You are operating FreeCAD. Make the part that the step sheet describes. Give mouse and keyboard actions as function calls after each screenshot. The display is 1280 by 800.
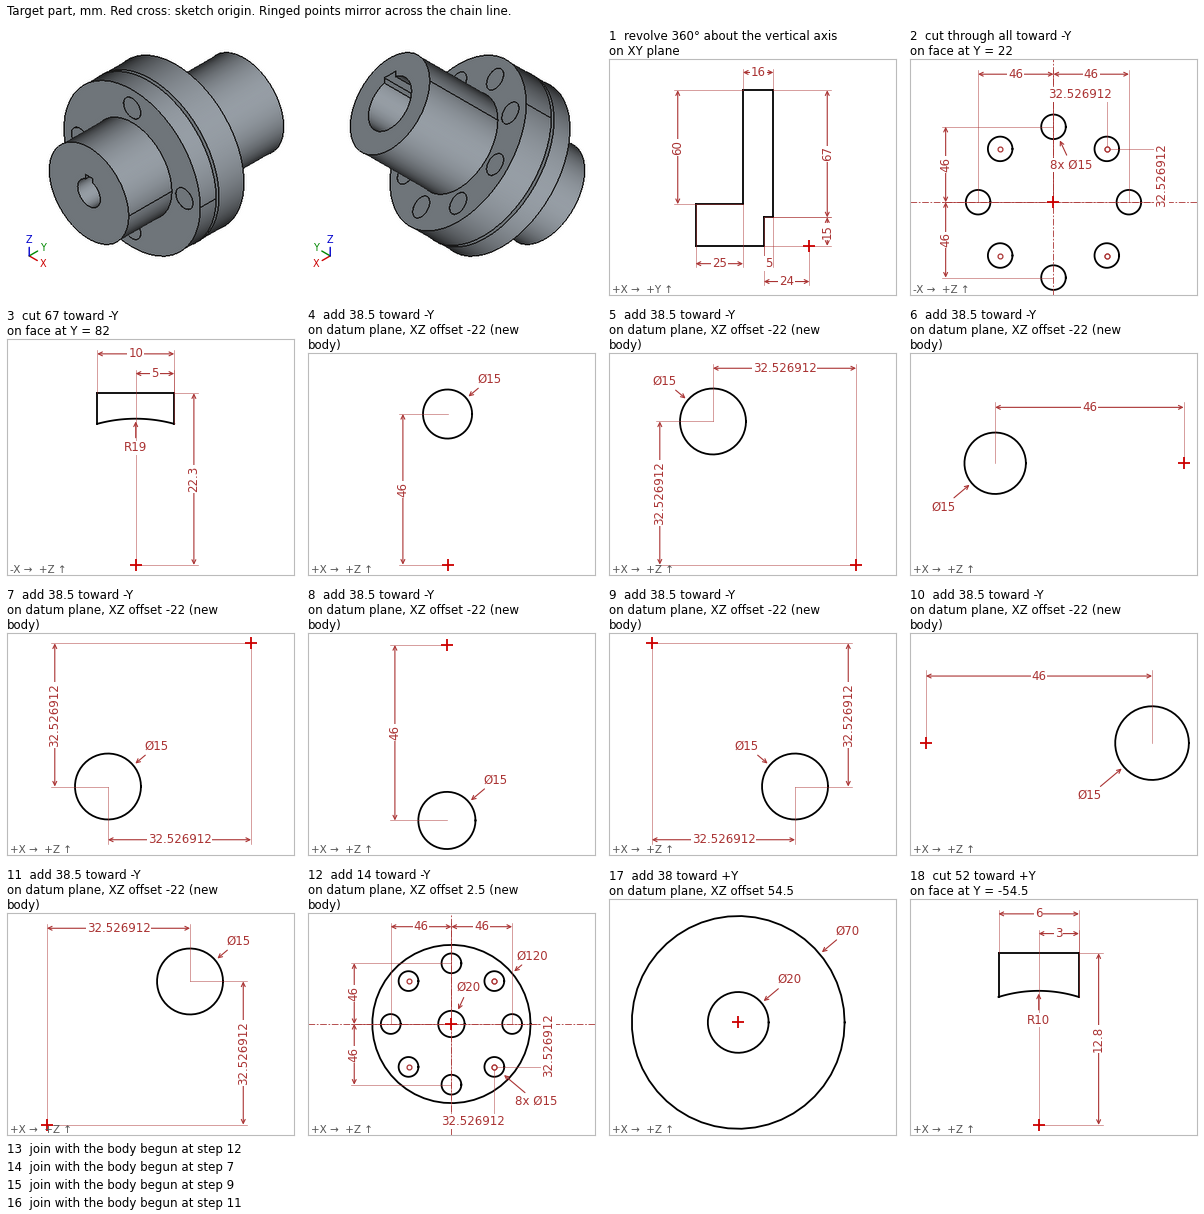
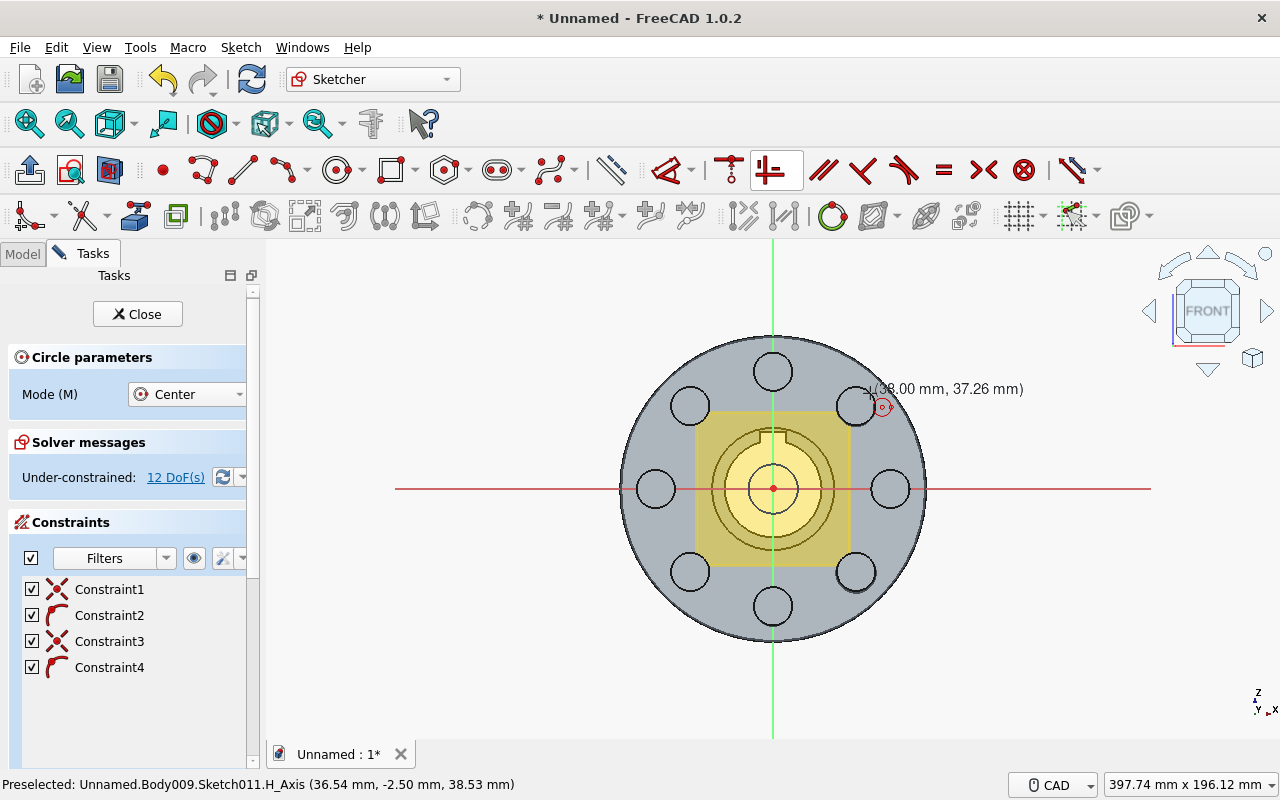
click(690, 572)
click(704, 558)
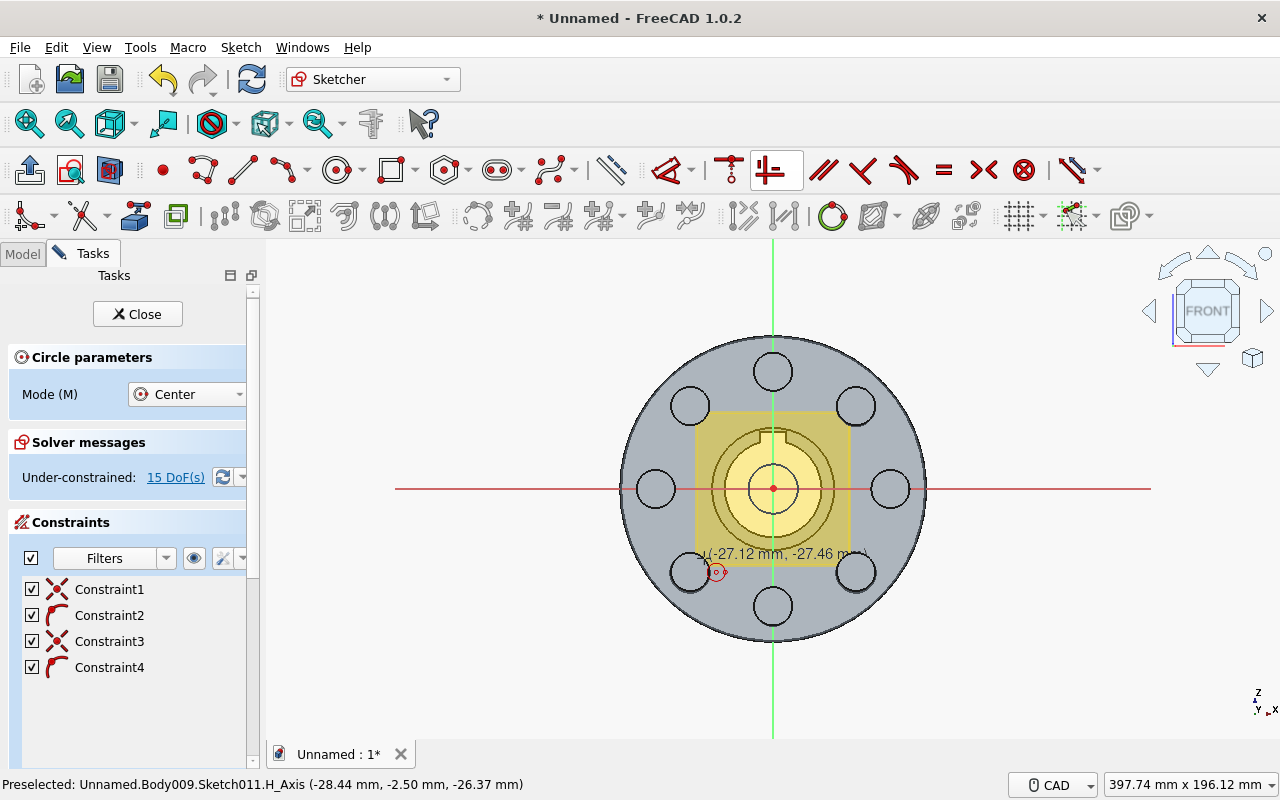
click(656, 489)
click(662, 471)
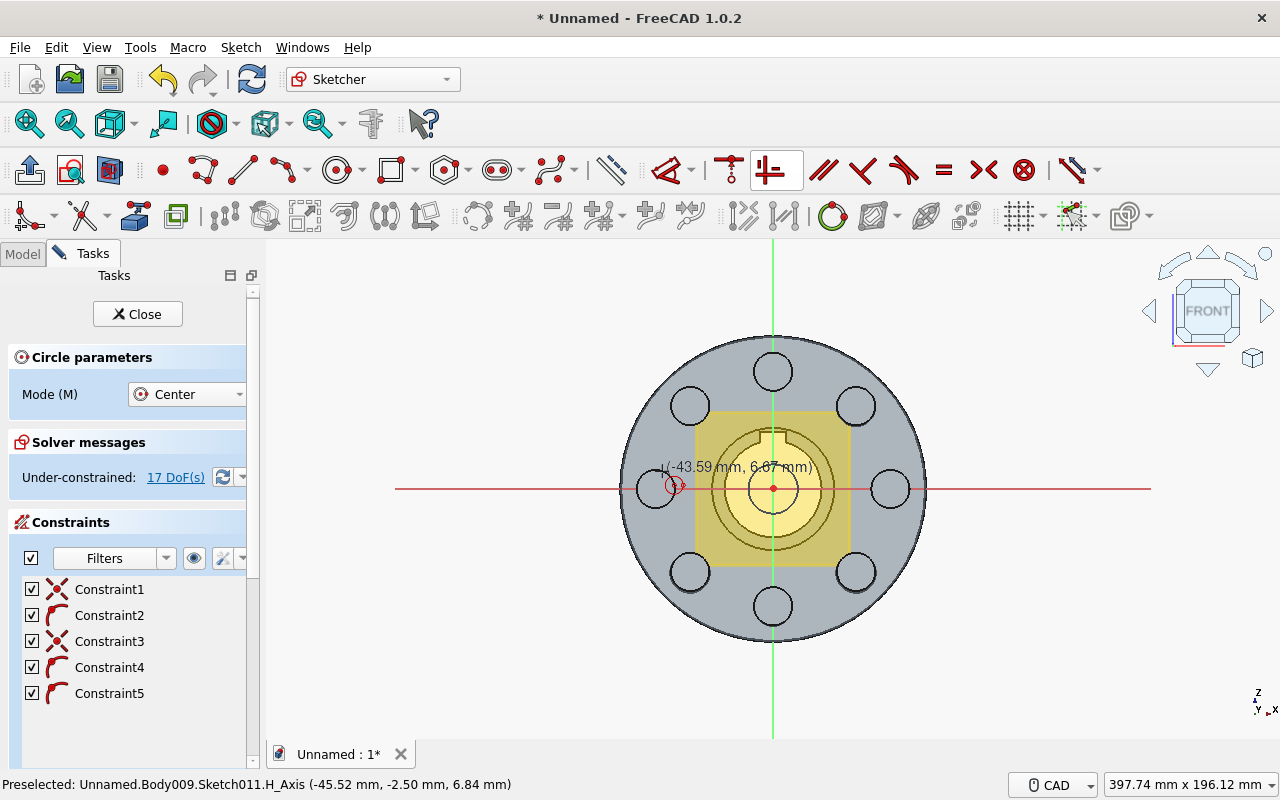
click(773, 372)
click(791, 365)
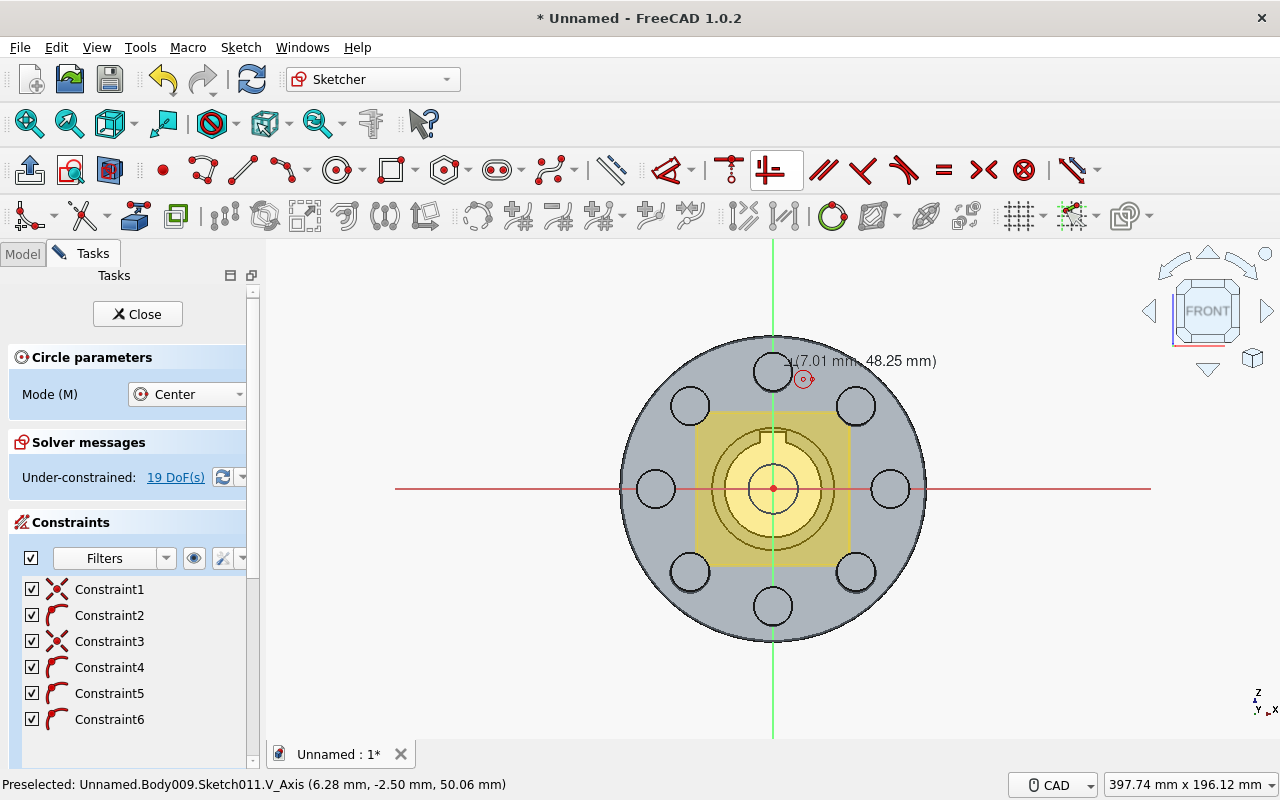
click(690, 406)
click(704, 393)
key(Escape)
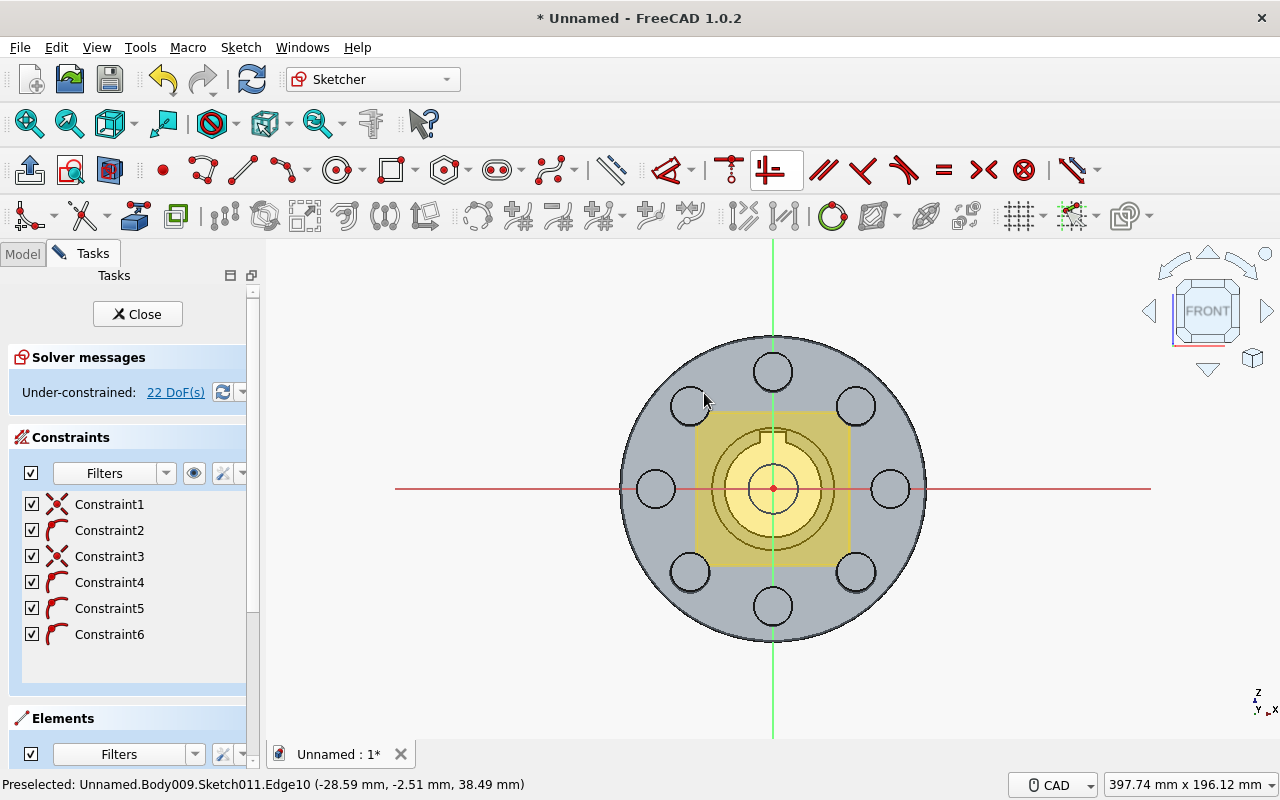
click(870, 559)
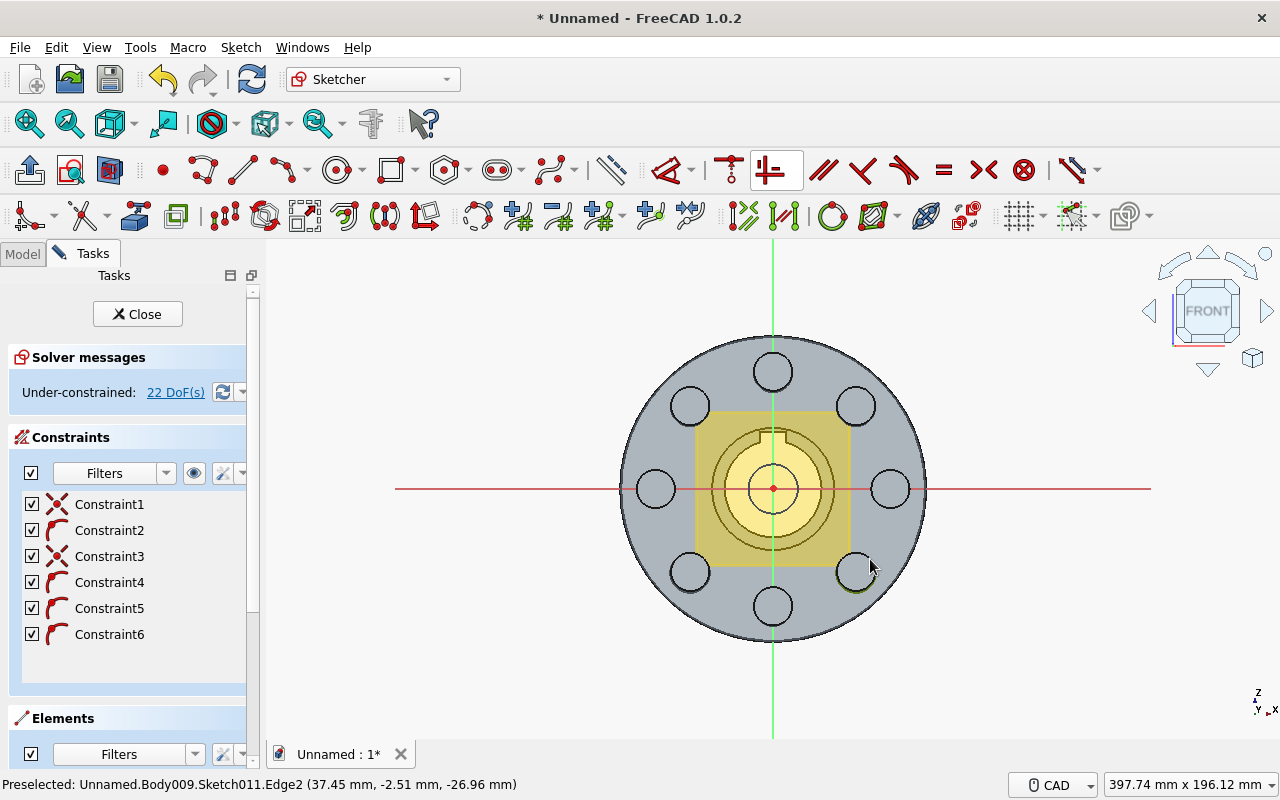
click(786, 594)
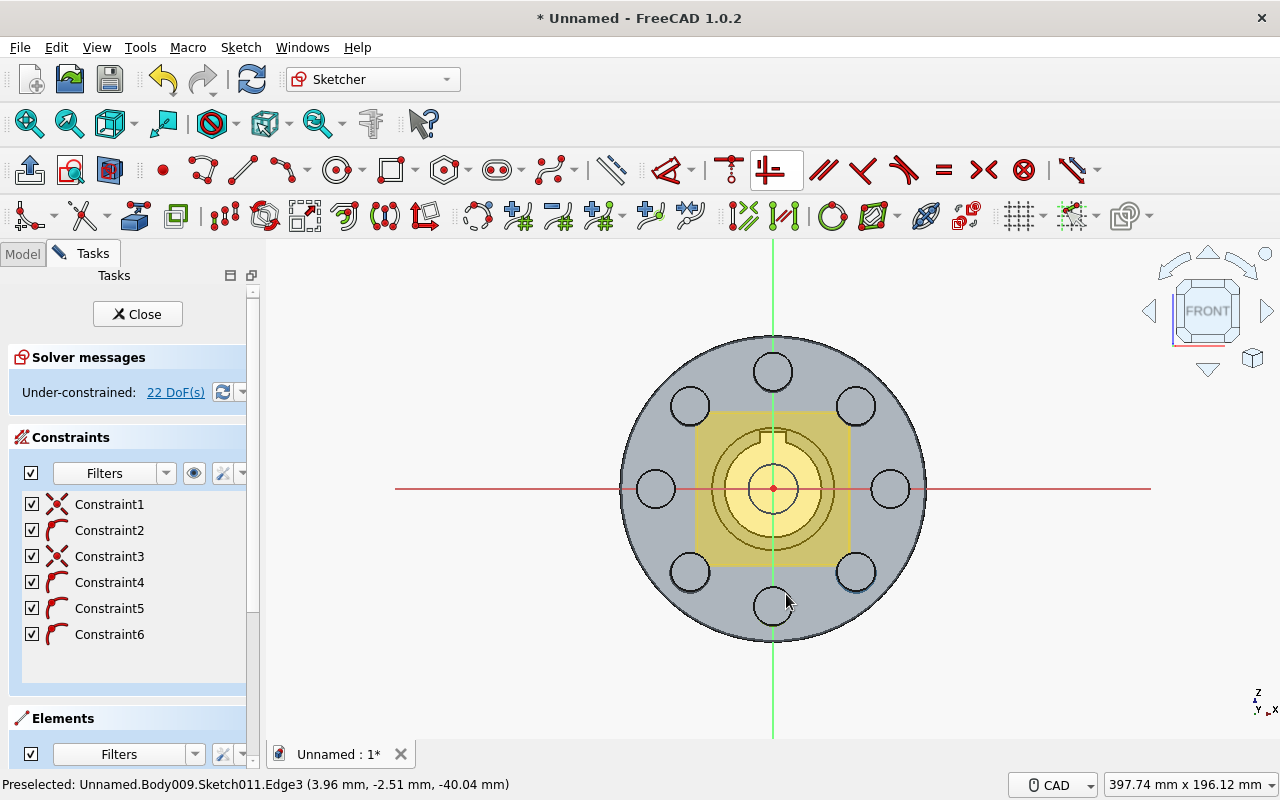
click(903, 476)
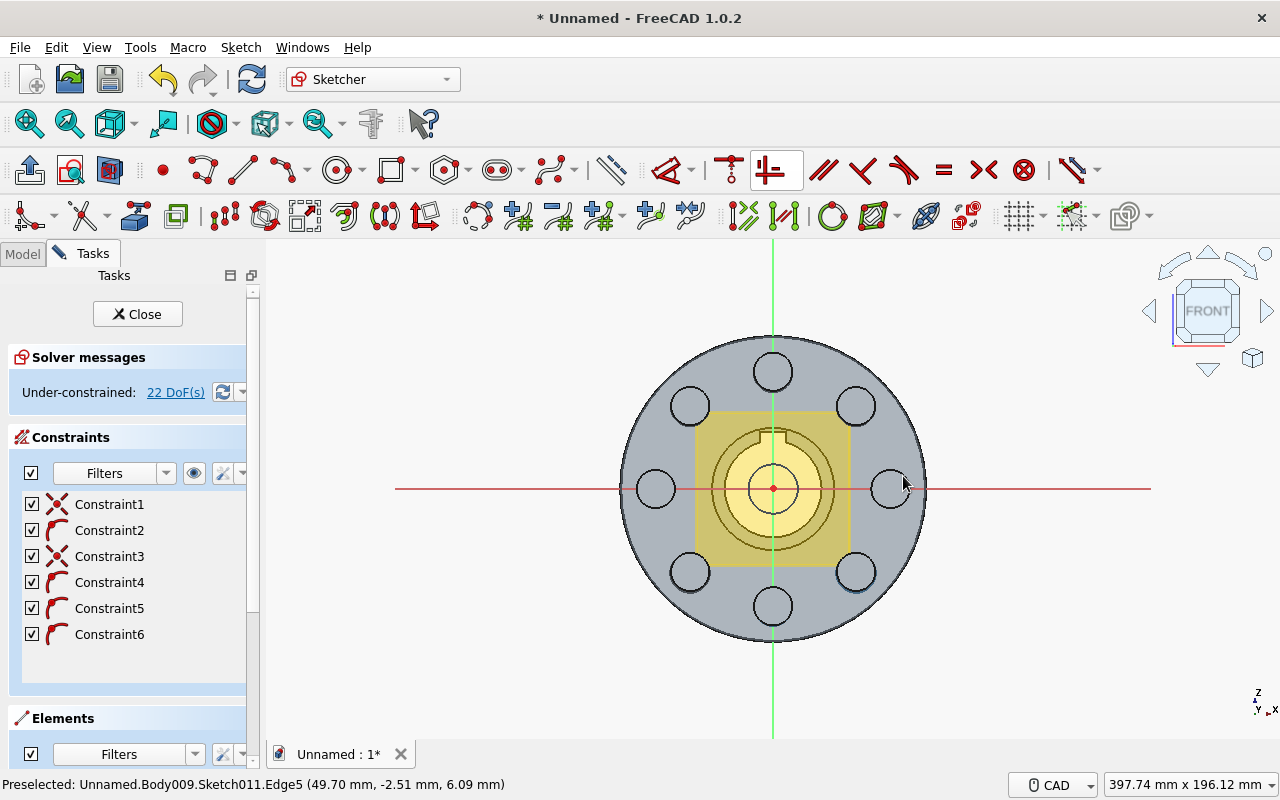
click(869, 393)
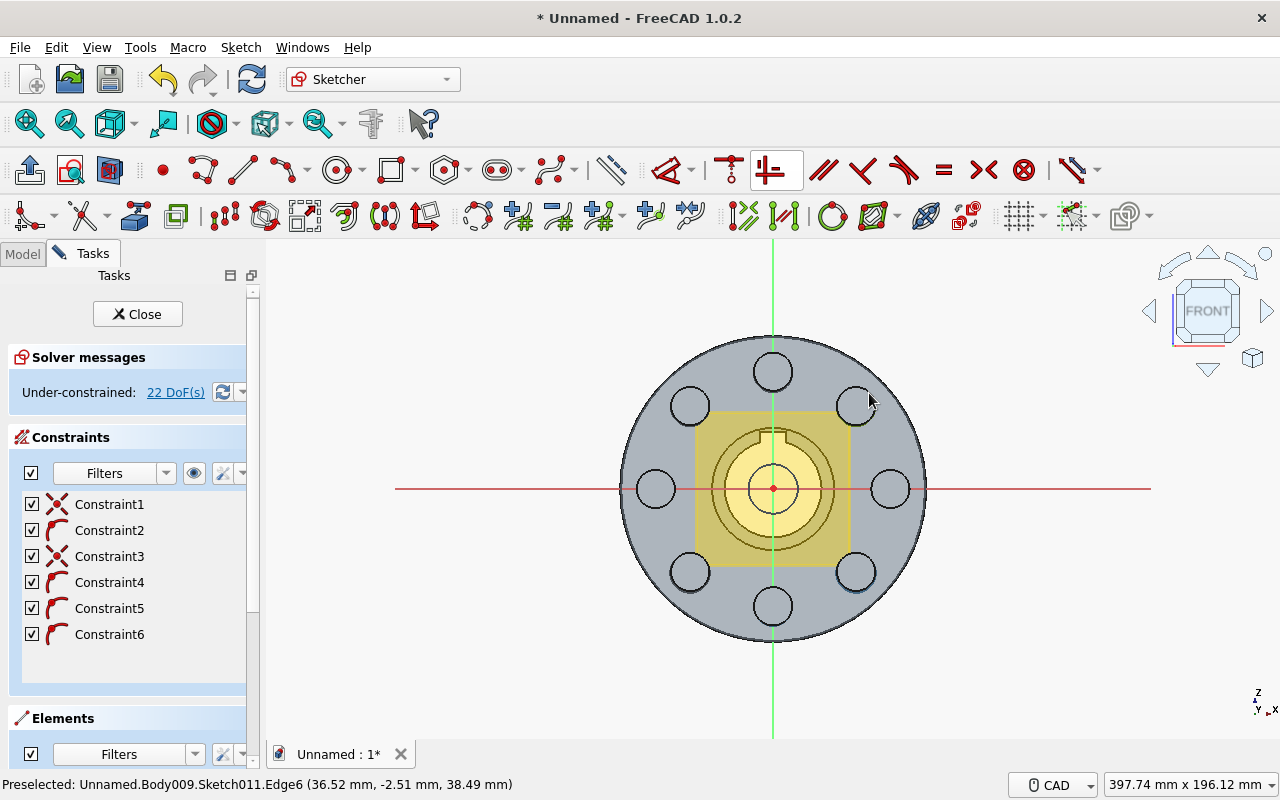
click(704, 559)